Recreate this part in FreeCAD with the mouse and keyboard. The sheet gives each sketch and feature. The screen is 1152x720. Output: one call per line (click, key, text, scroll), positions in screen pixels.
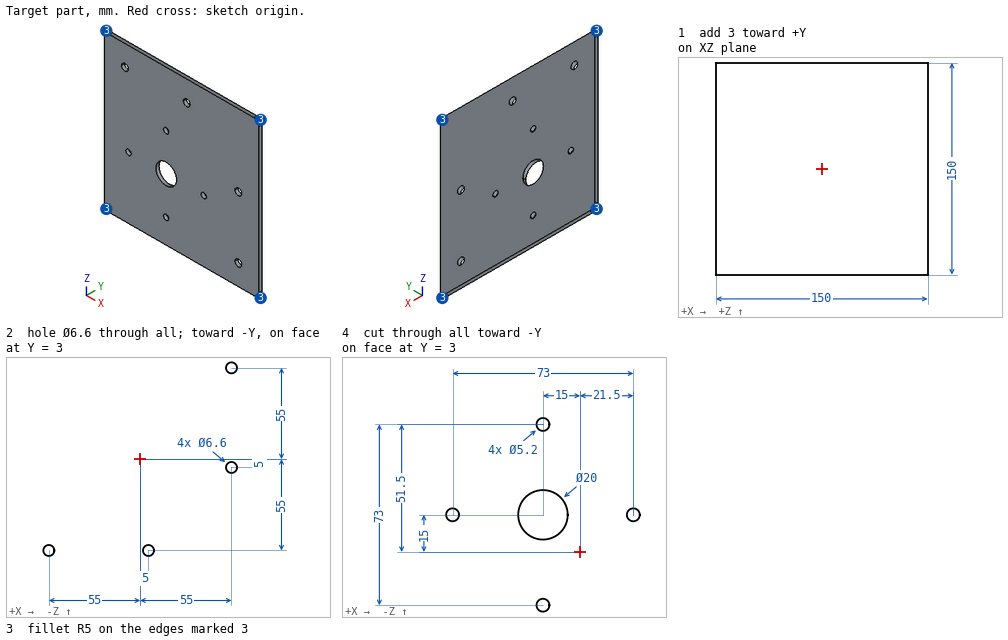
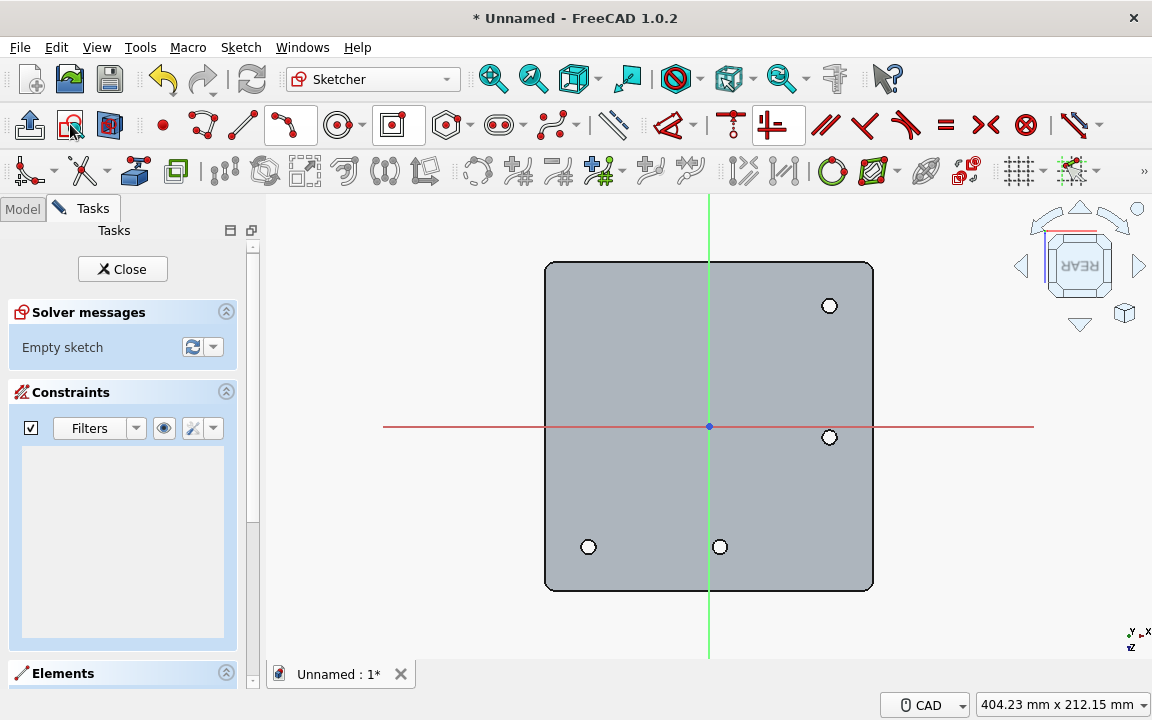
scroll(719, 354, up, 3)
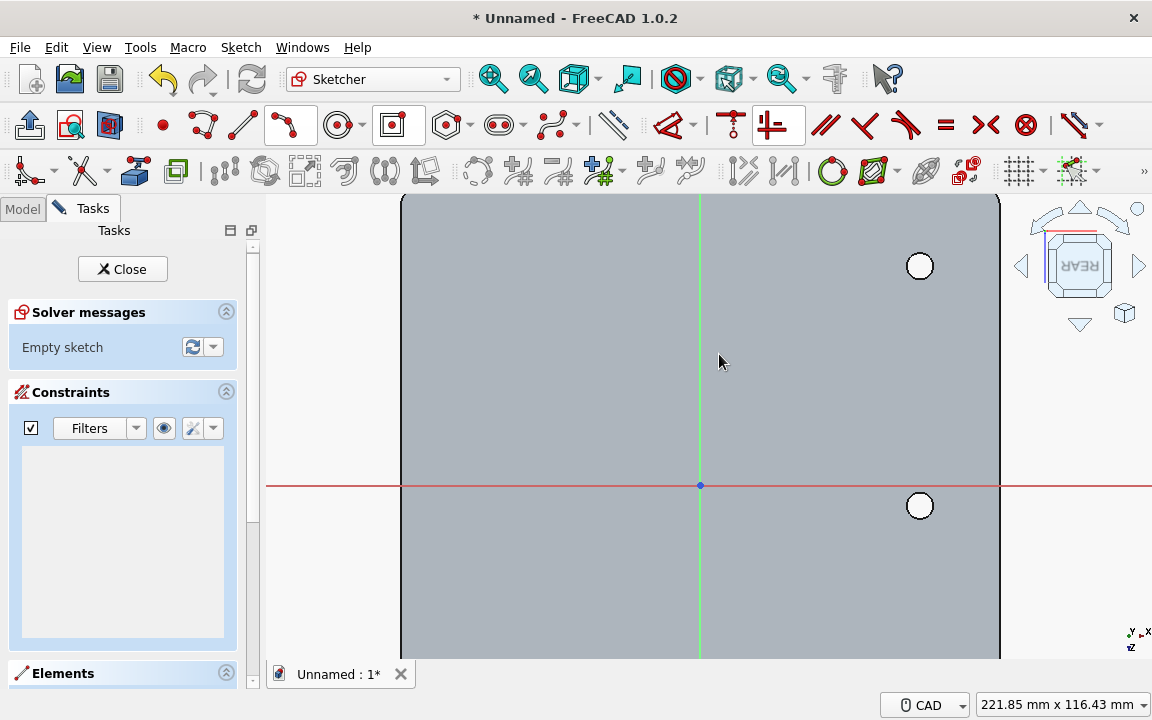
click(338, 126)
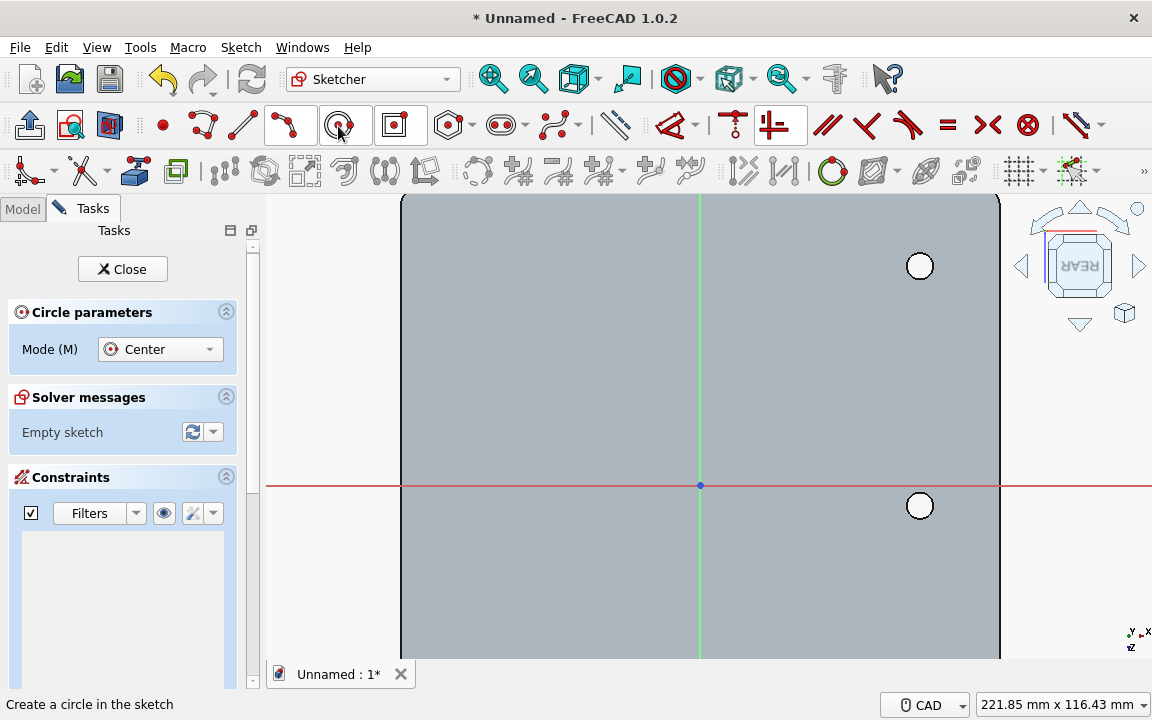
click(640, 426)
click(669, 398)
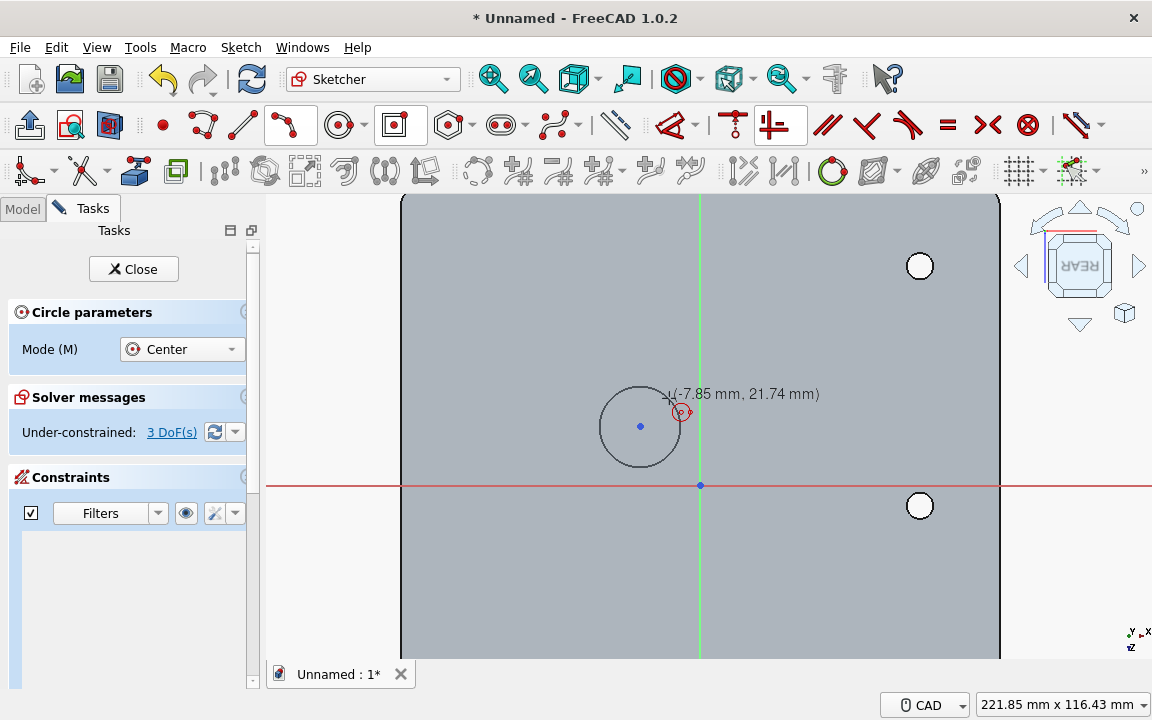
scroll(640, 280, up, 4)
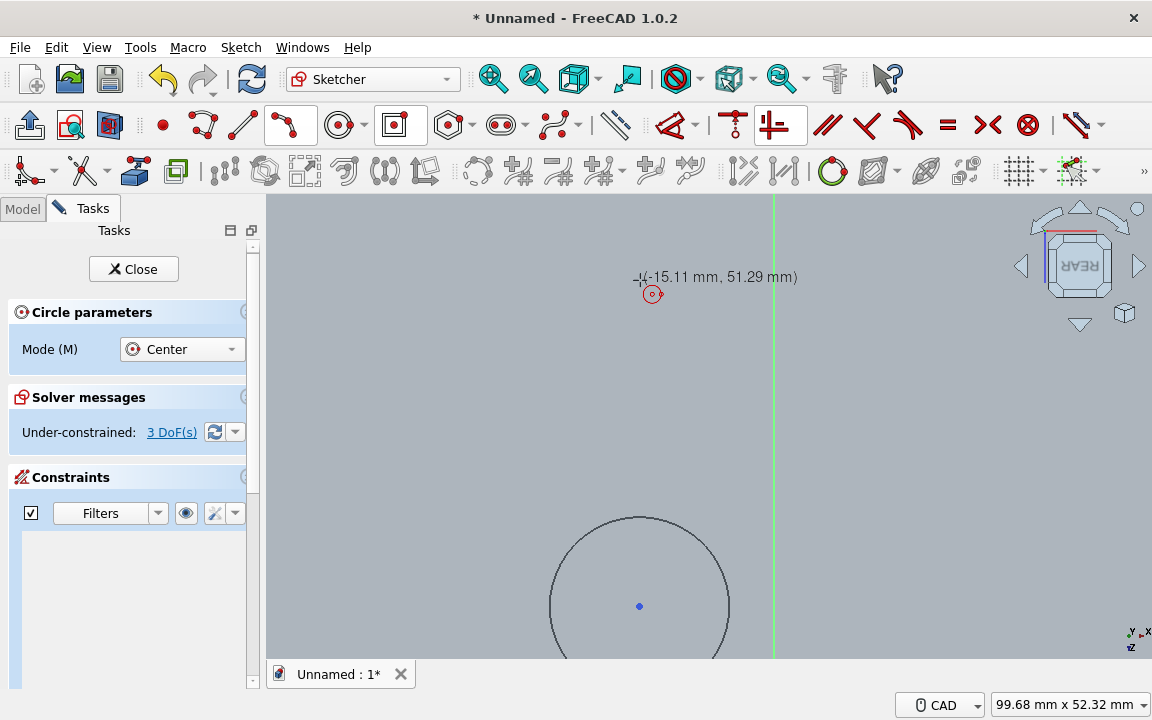
click(640, 280)
click(657, 264)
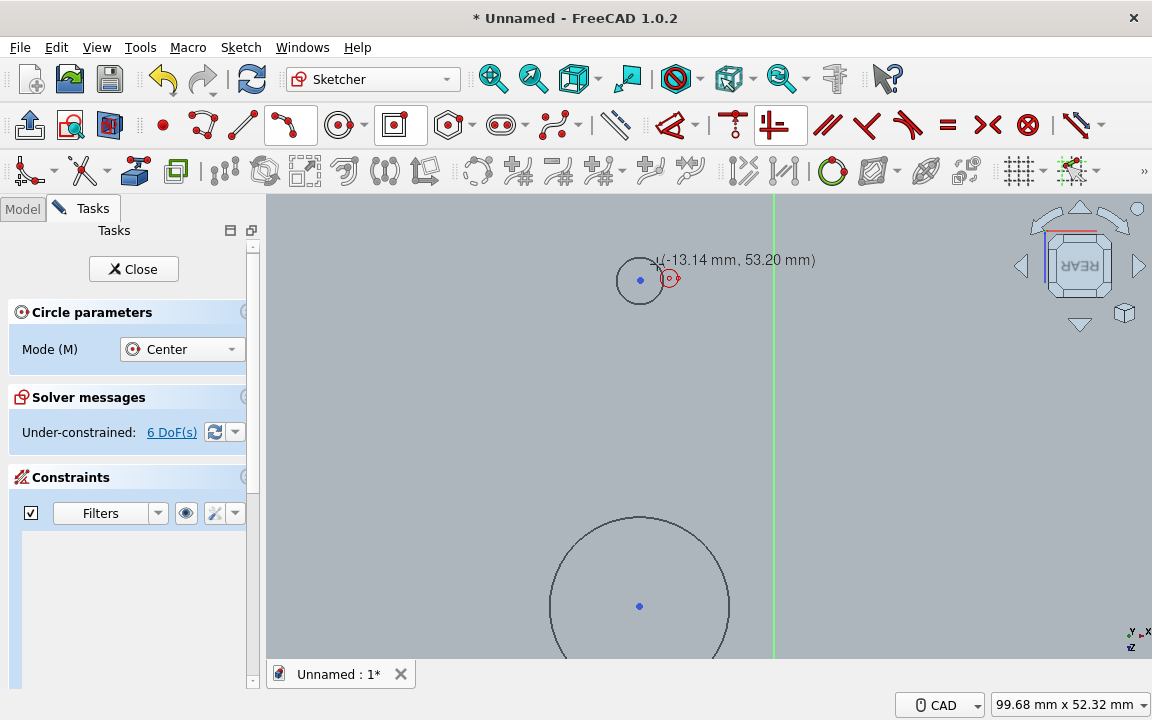
click(965, 605)
click(981, 588)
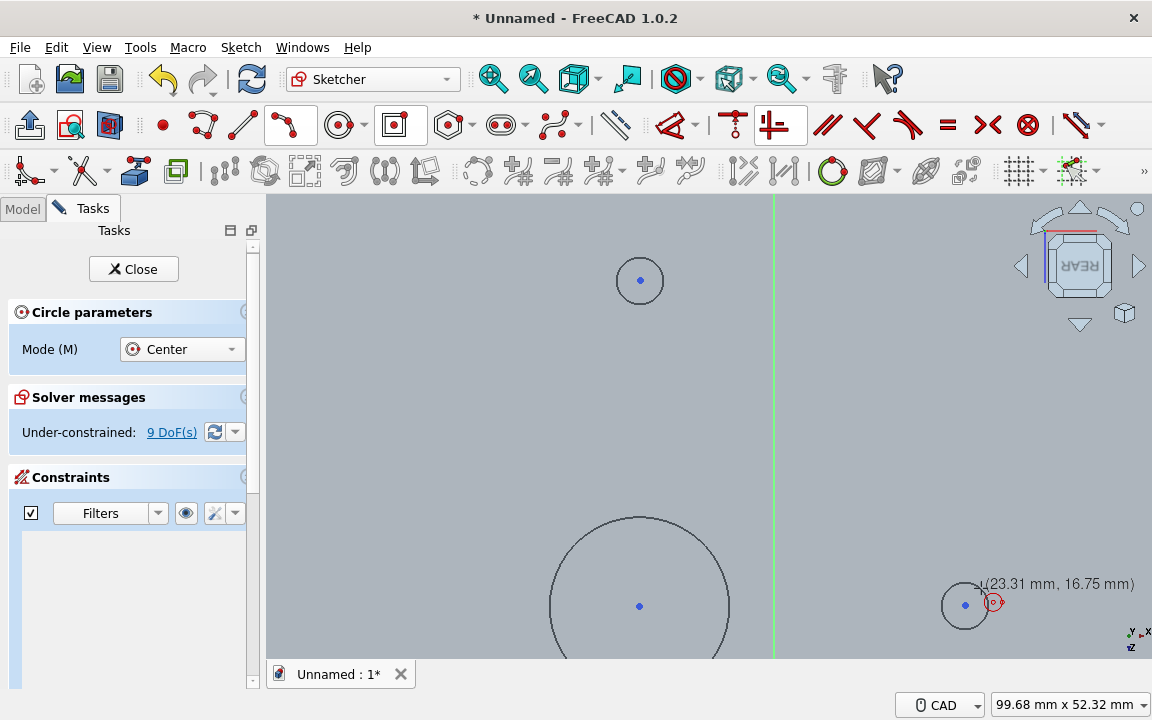
scroll(641, 281, down, 4)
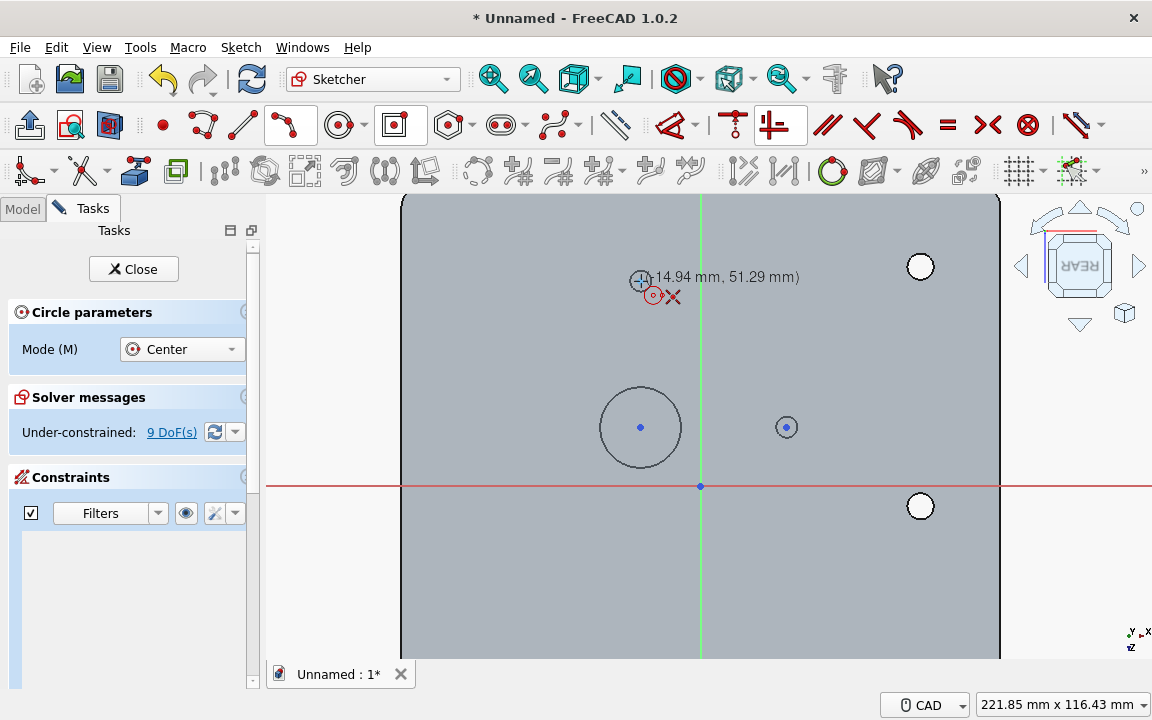
scroll(641, 572, up, 4)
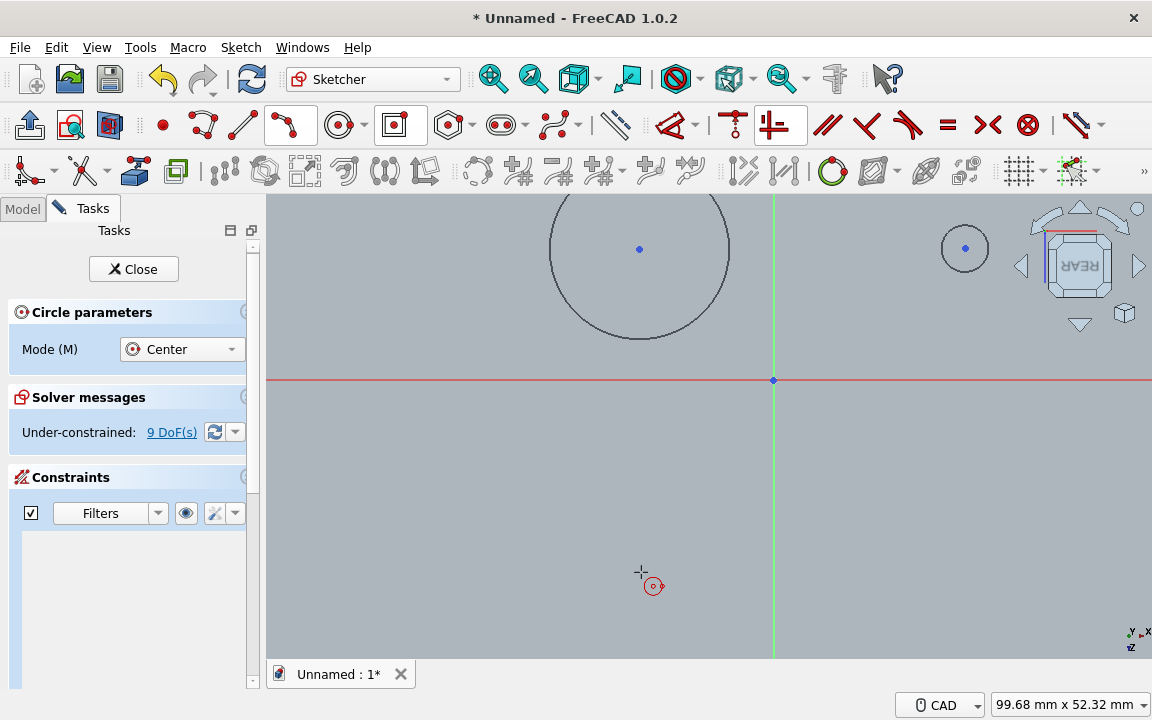
click(640, 572)
click(657, 555)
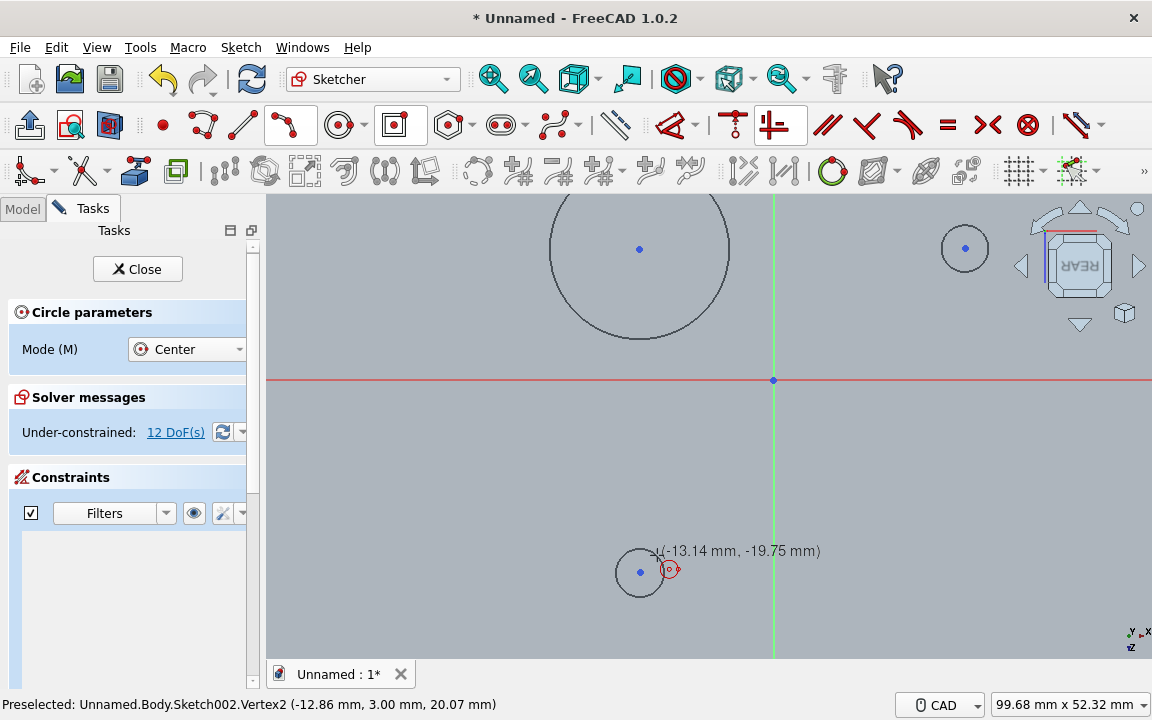
click(316, 247)
click(332, 231)
key(Escape)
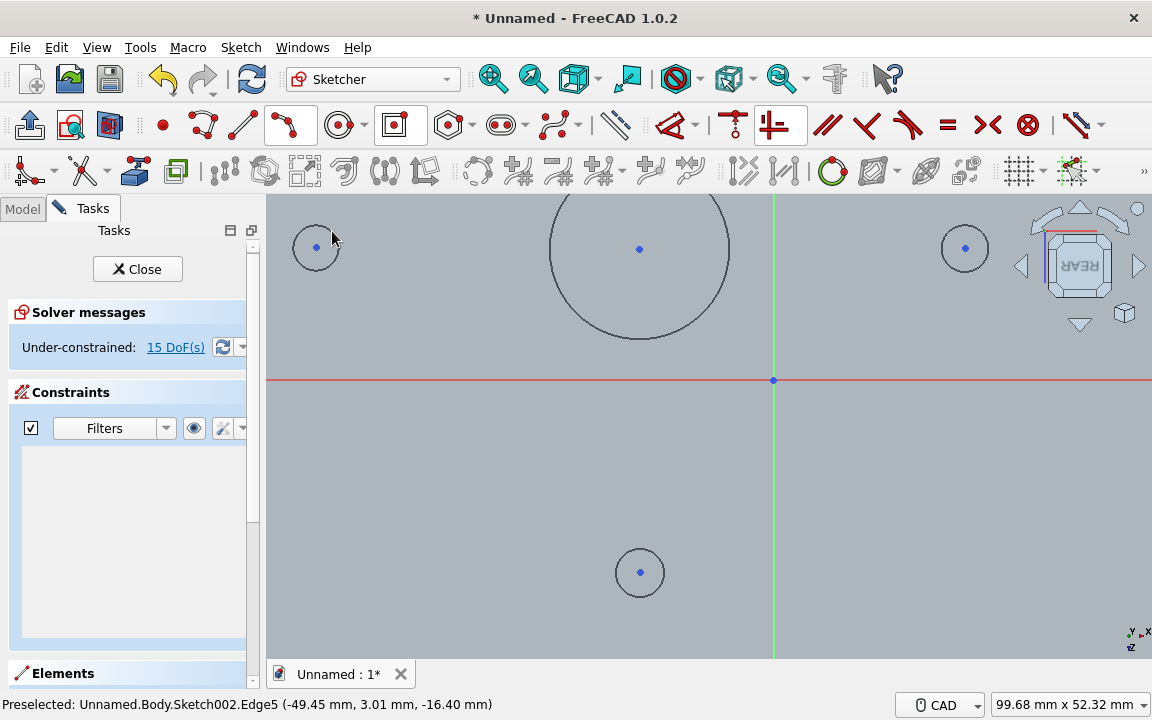
scroll(641, 573, down, 4)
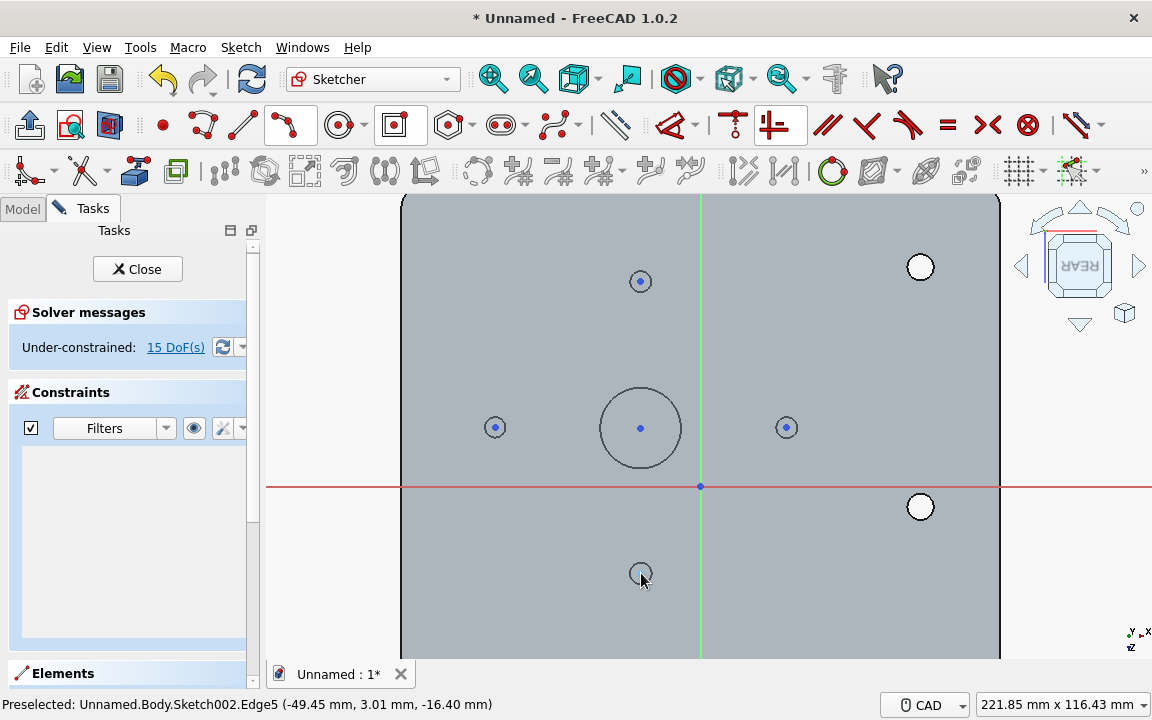
scroll(648, 274, up, 2)